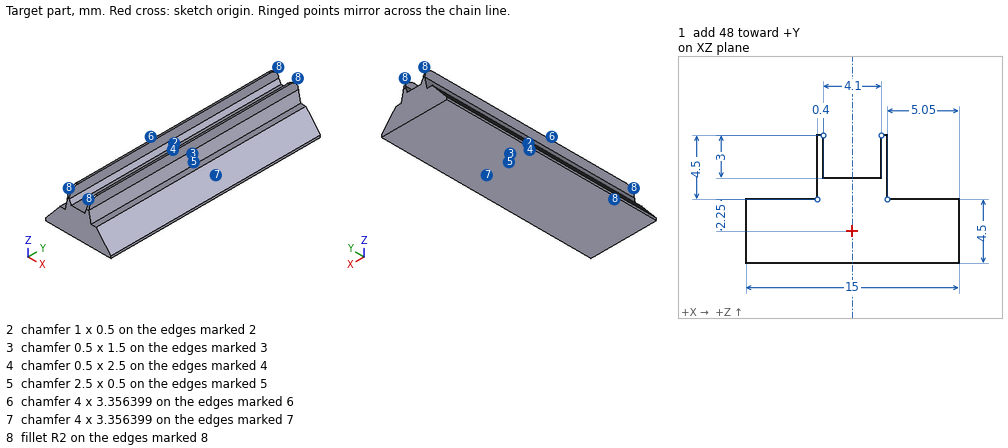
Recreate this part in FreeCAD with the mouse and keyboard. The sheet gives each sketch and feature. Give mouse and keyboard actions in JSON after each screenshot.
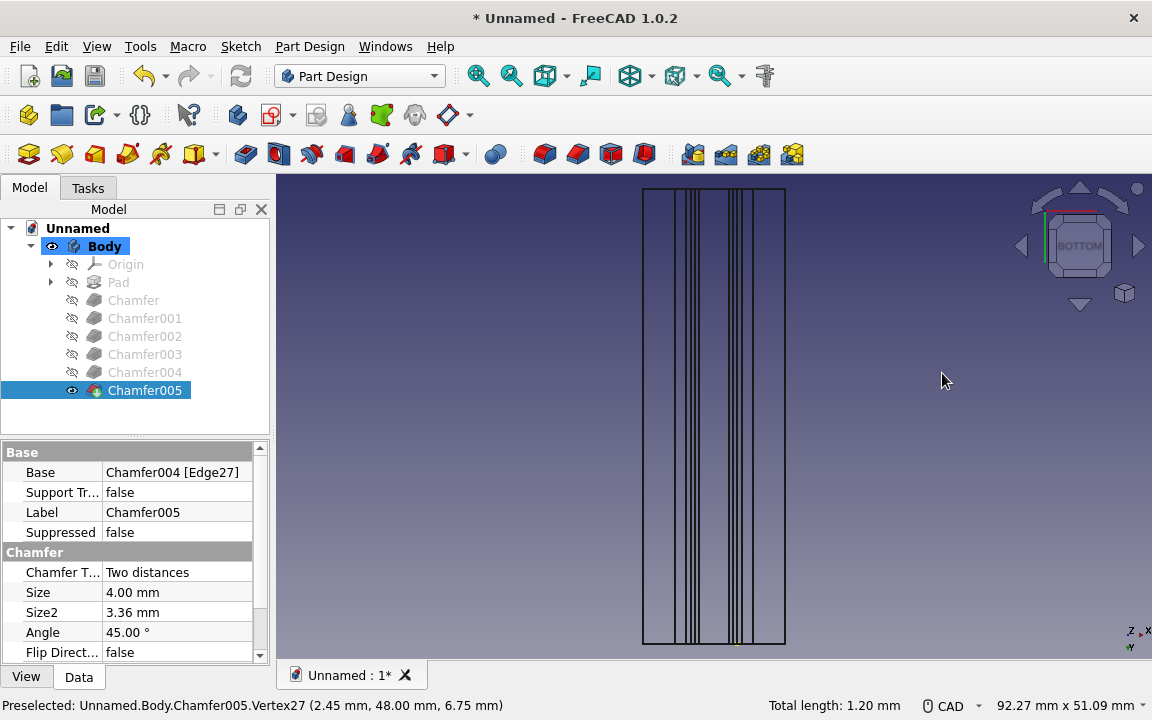
{"action": "key", "text": "4"}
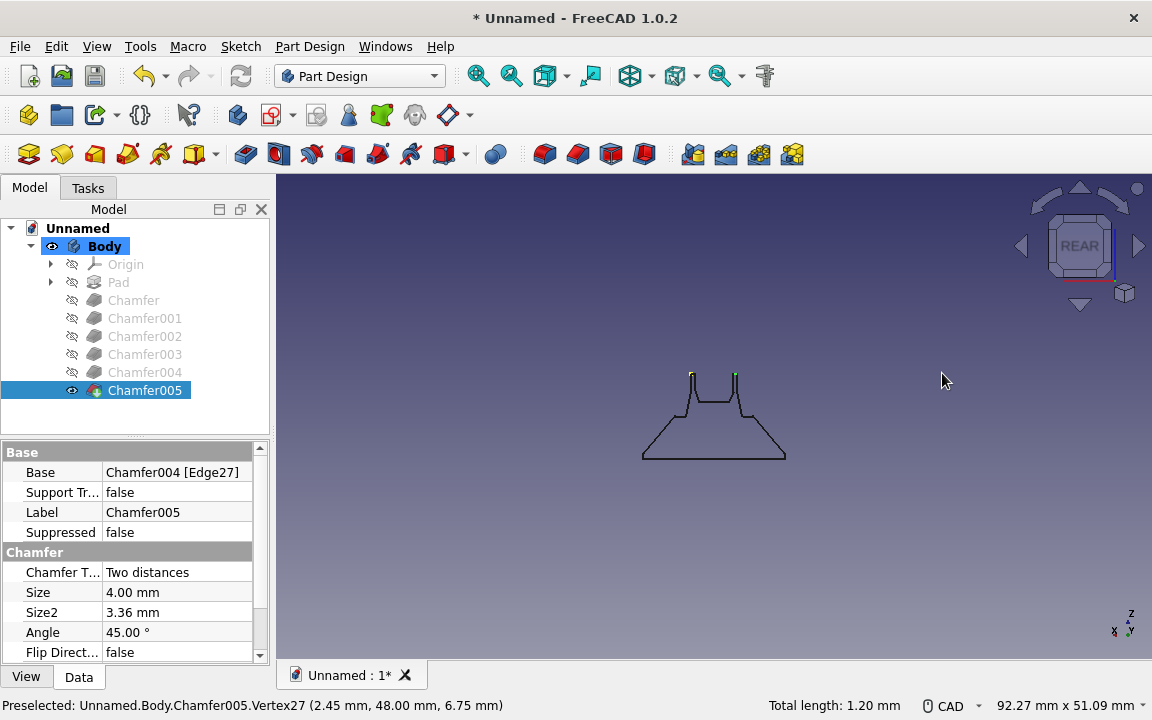
{"action": "left_click", "coordinate": [479, 76]}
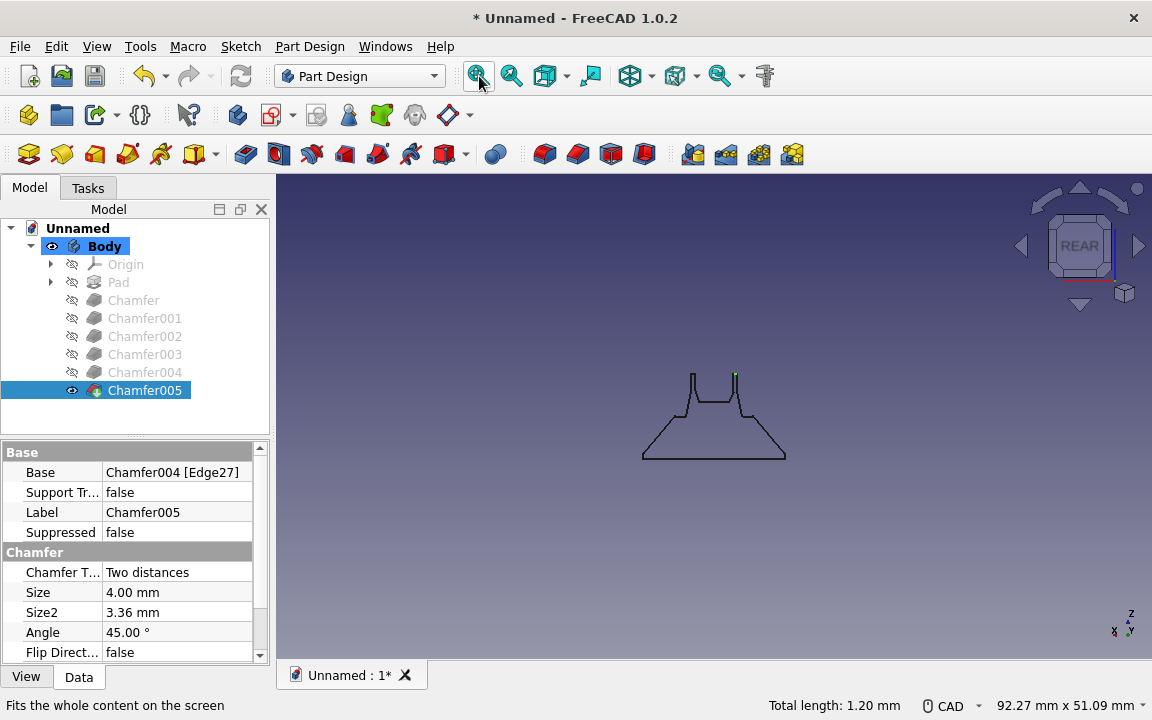
{"action": "scroll", "coordinate": [693, 373], "scroll_direction": "up", "scroll_amount": 12}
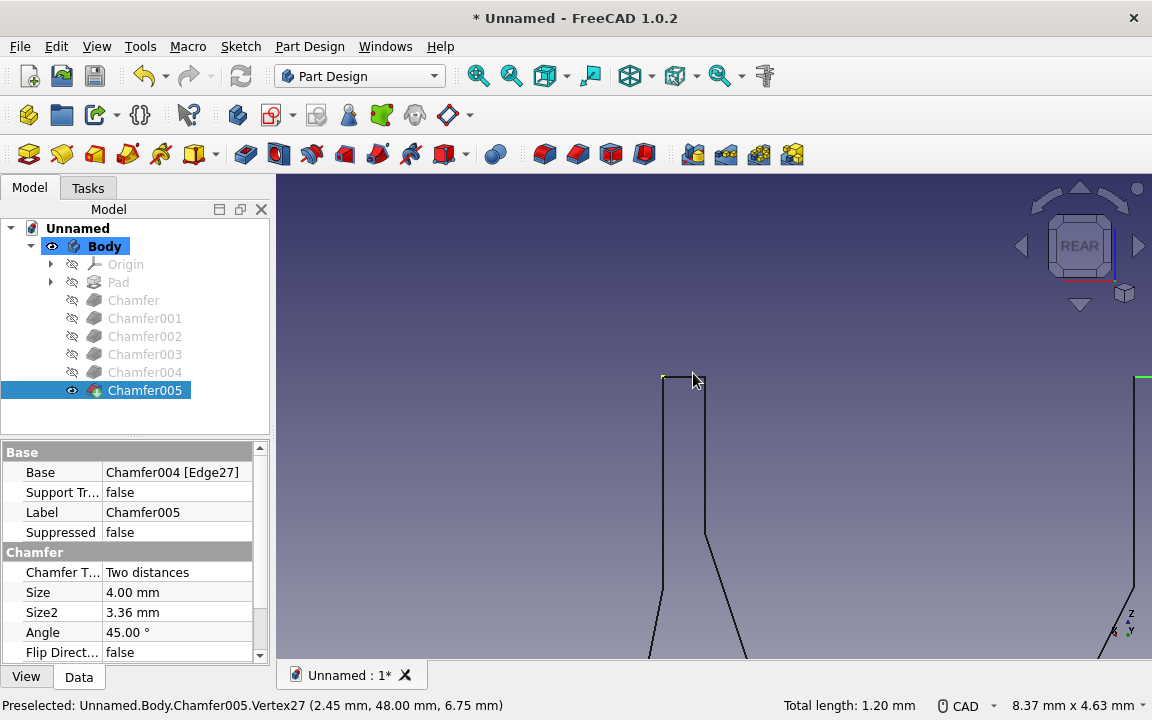
{"action": "left_click", "coordinate": [684, 376], "text": "ctrl"}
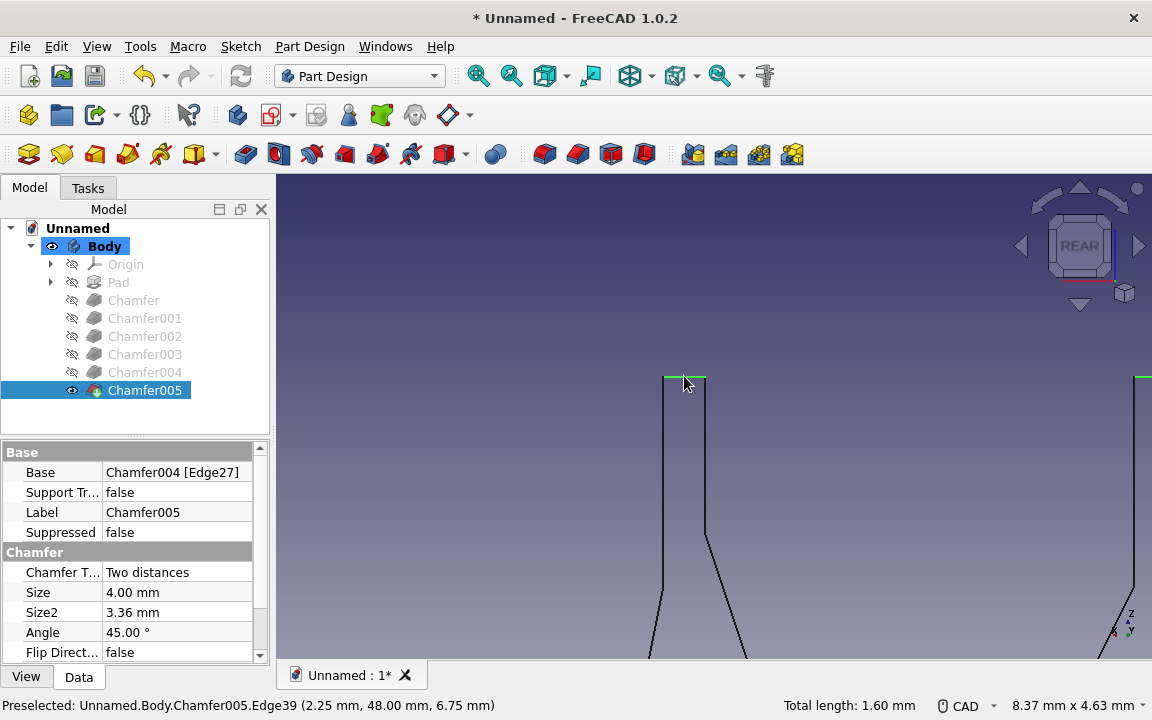
{"action": "key", "text": "v 1"}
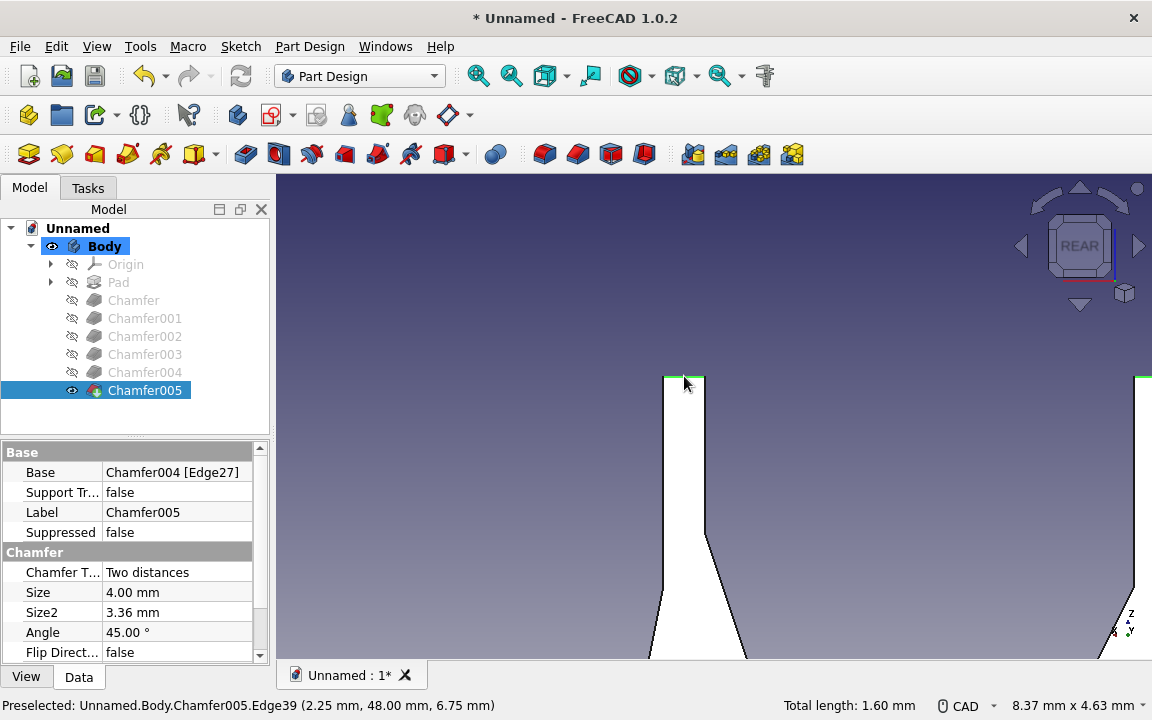
{"action": "left_click", "coordinate": [545, 154]}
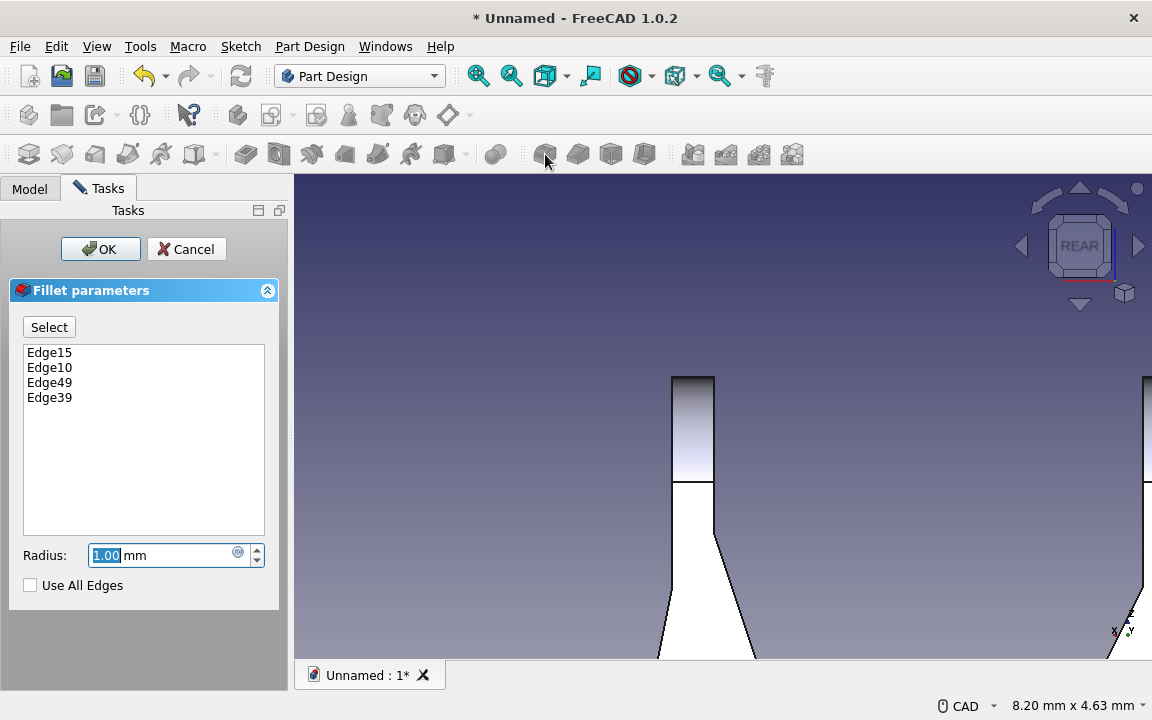
{"action": "type", "text": "2"}
{"action": "key", "text": "Tab"}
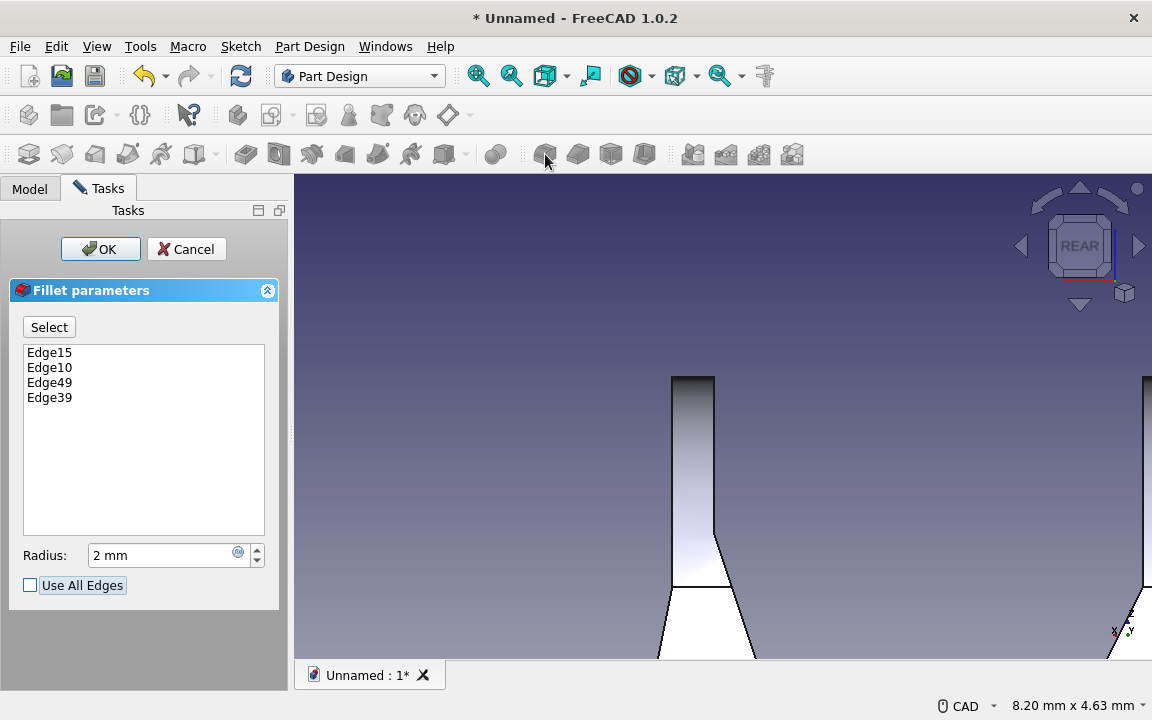
{"action": "left_click", "coordinate": [101, 249]}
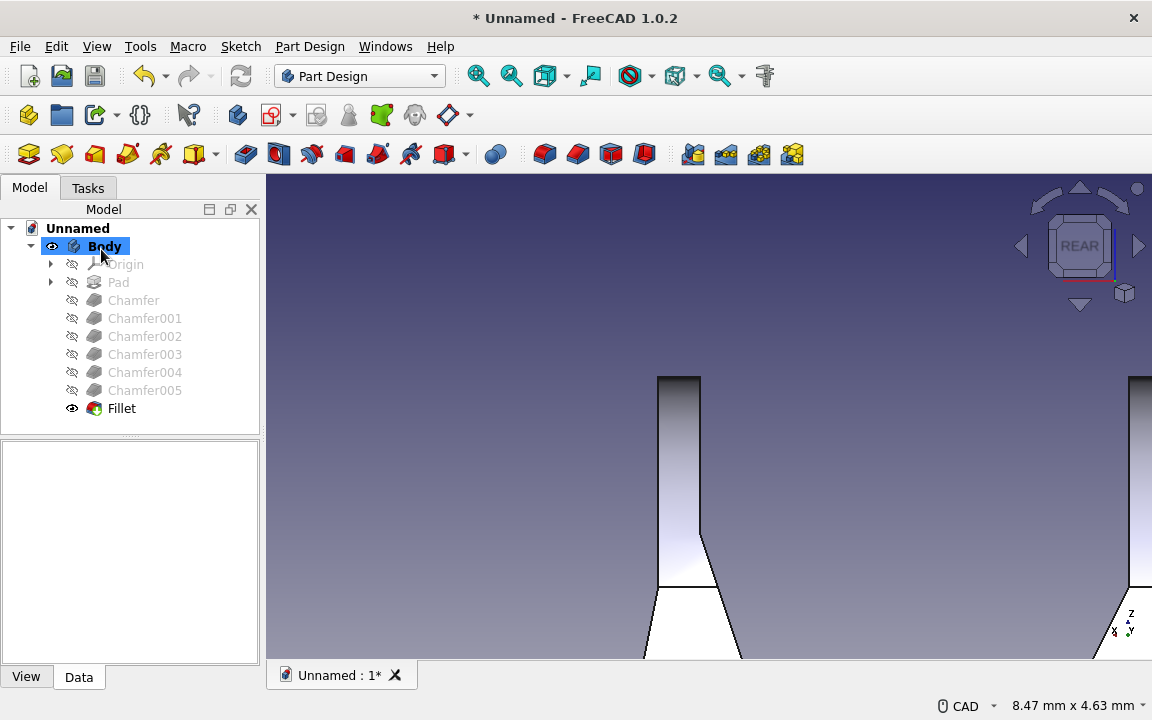
{"action": "key", "text": "0"}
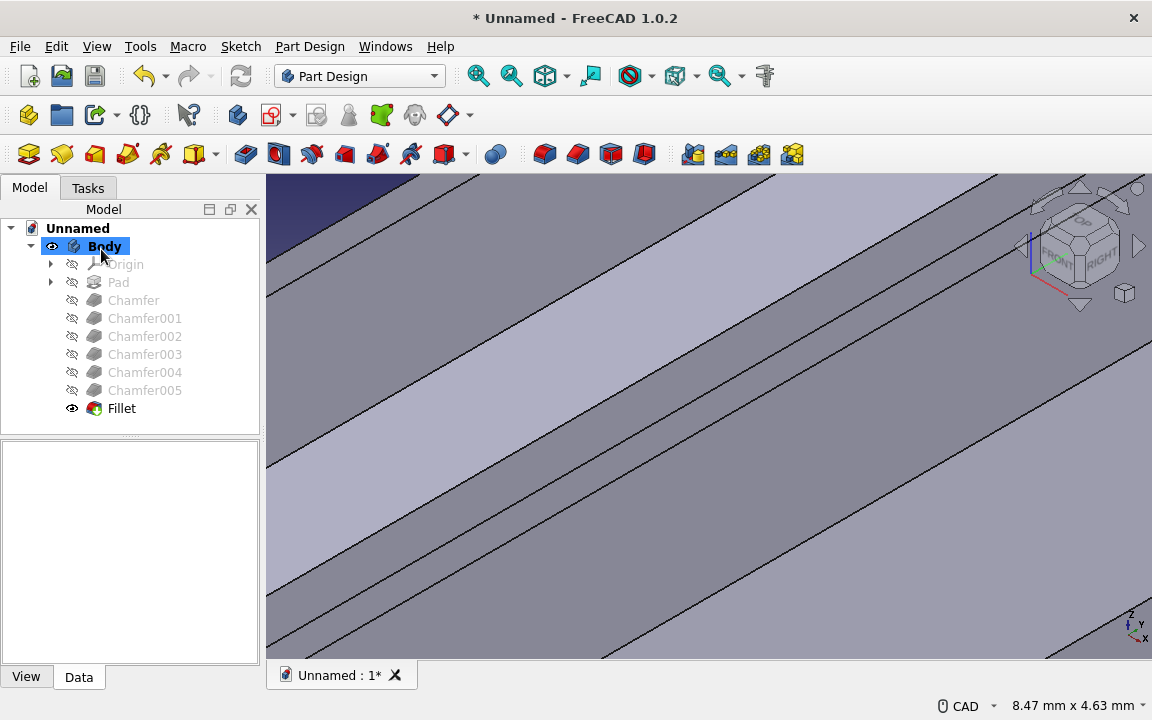
{"action": "left_click", "coordinate": [479, 76]}